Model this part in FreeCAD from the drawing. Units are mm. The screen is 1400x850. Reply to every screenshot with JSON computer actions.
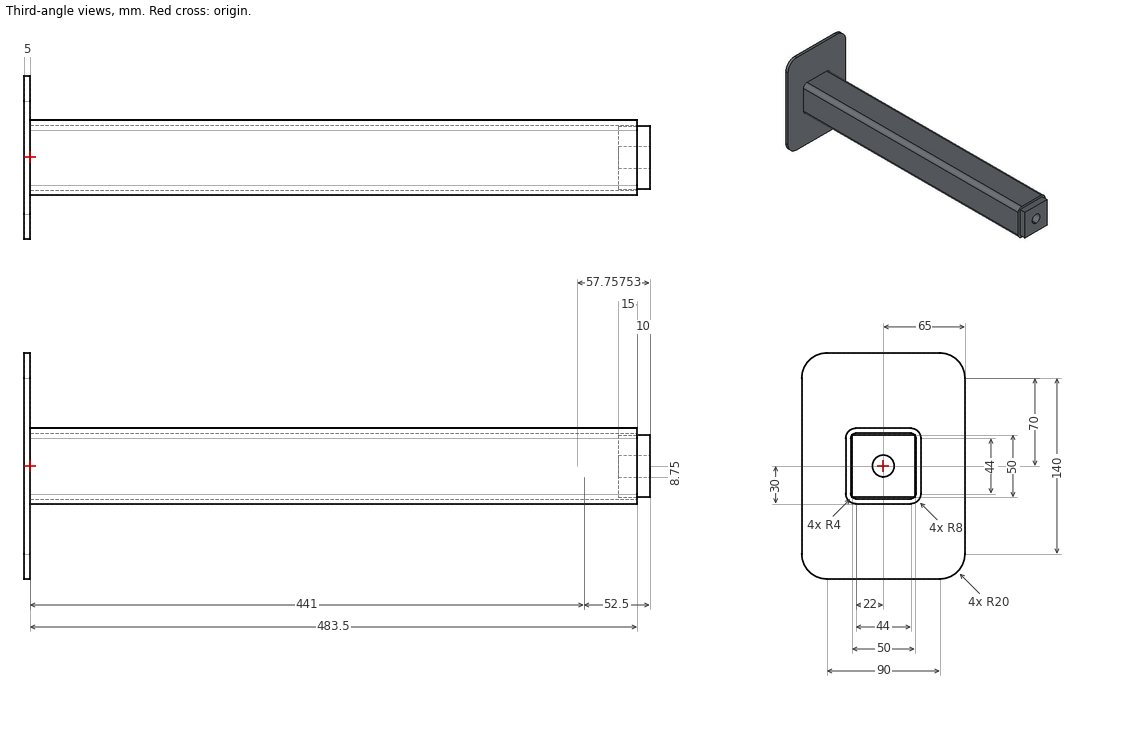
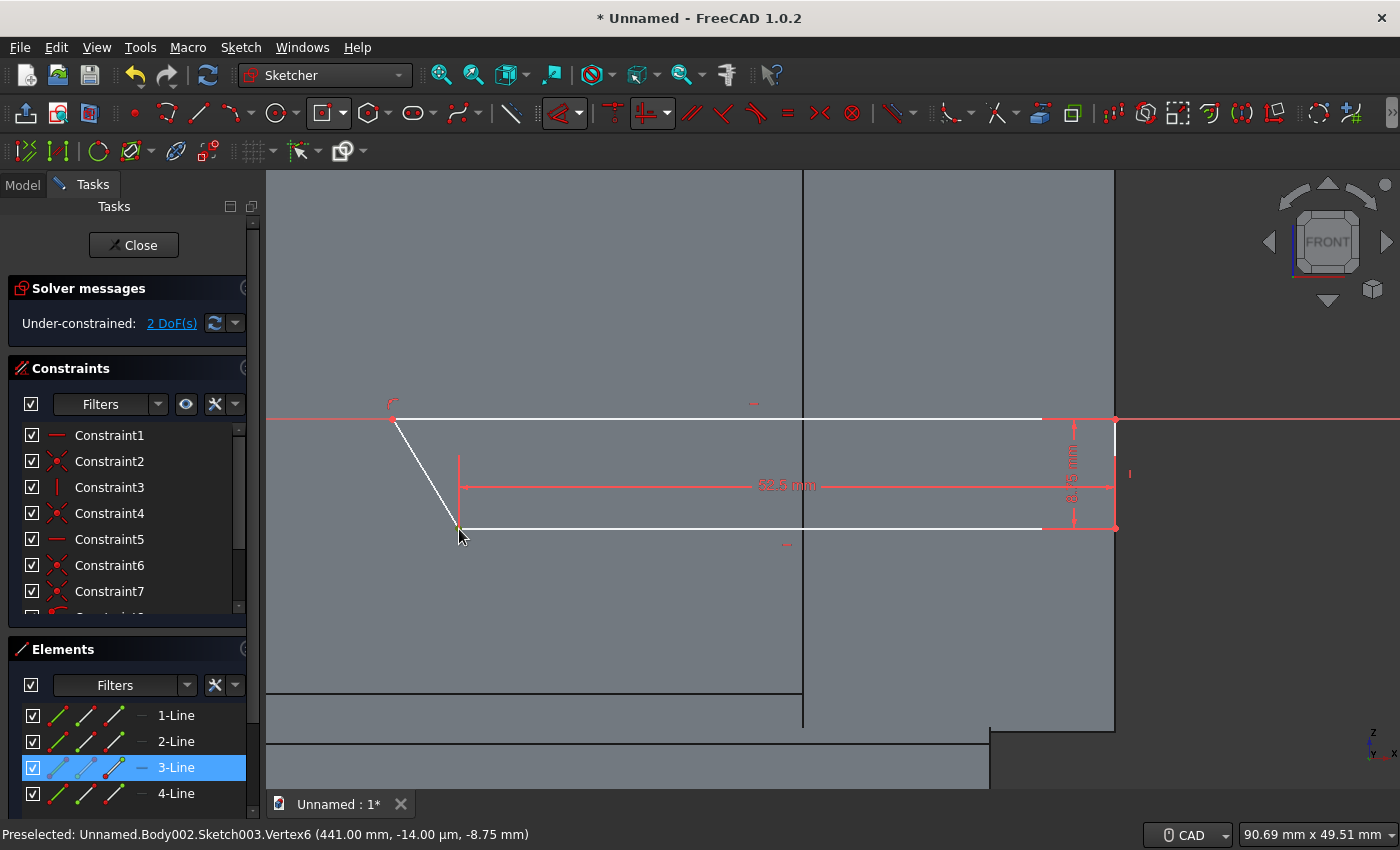
{"action": "left_click", "coordinate": [582, 114]}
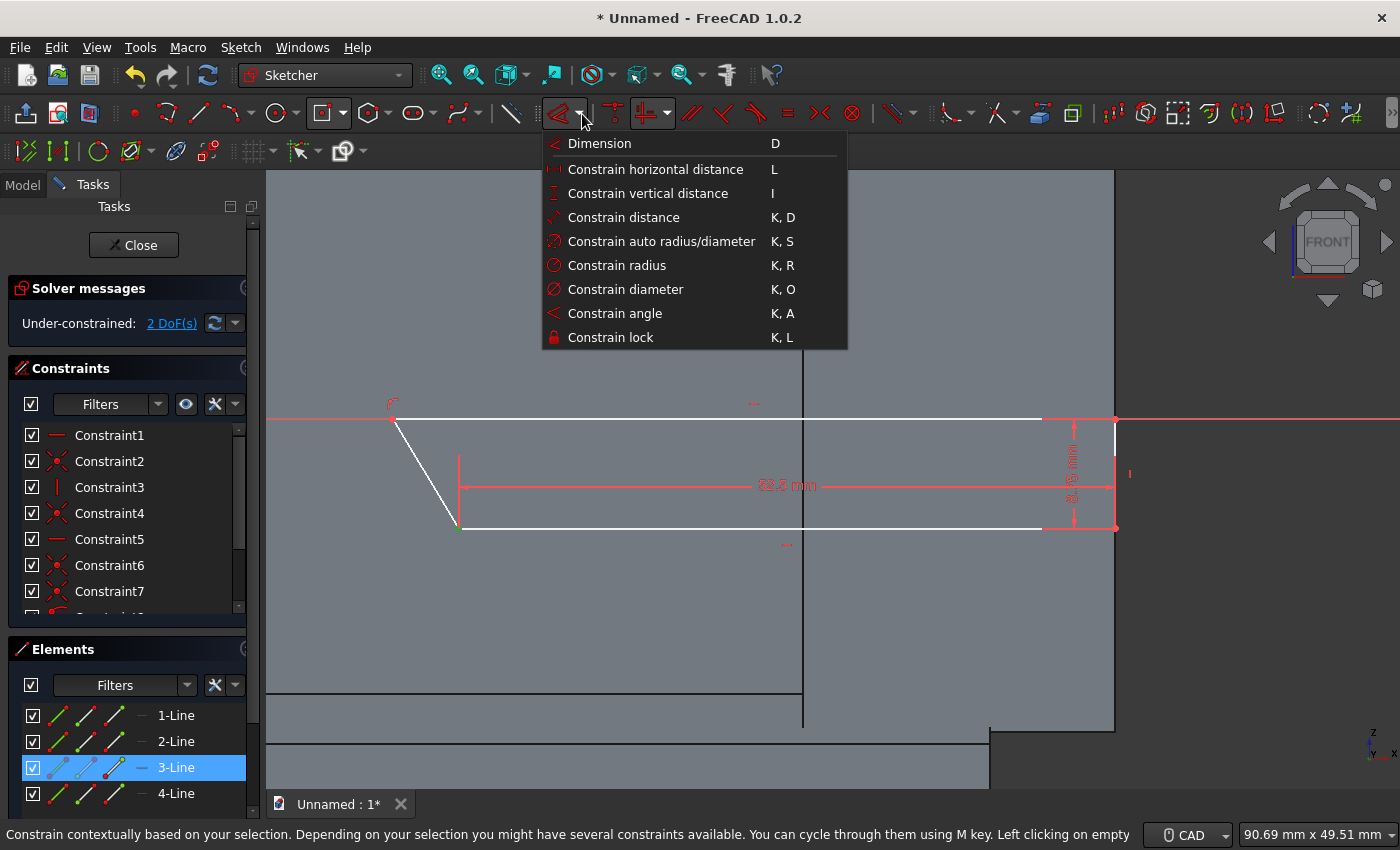
{"action": "left_click", "coordinate": [695, 169]}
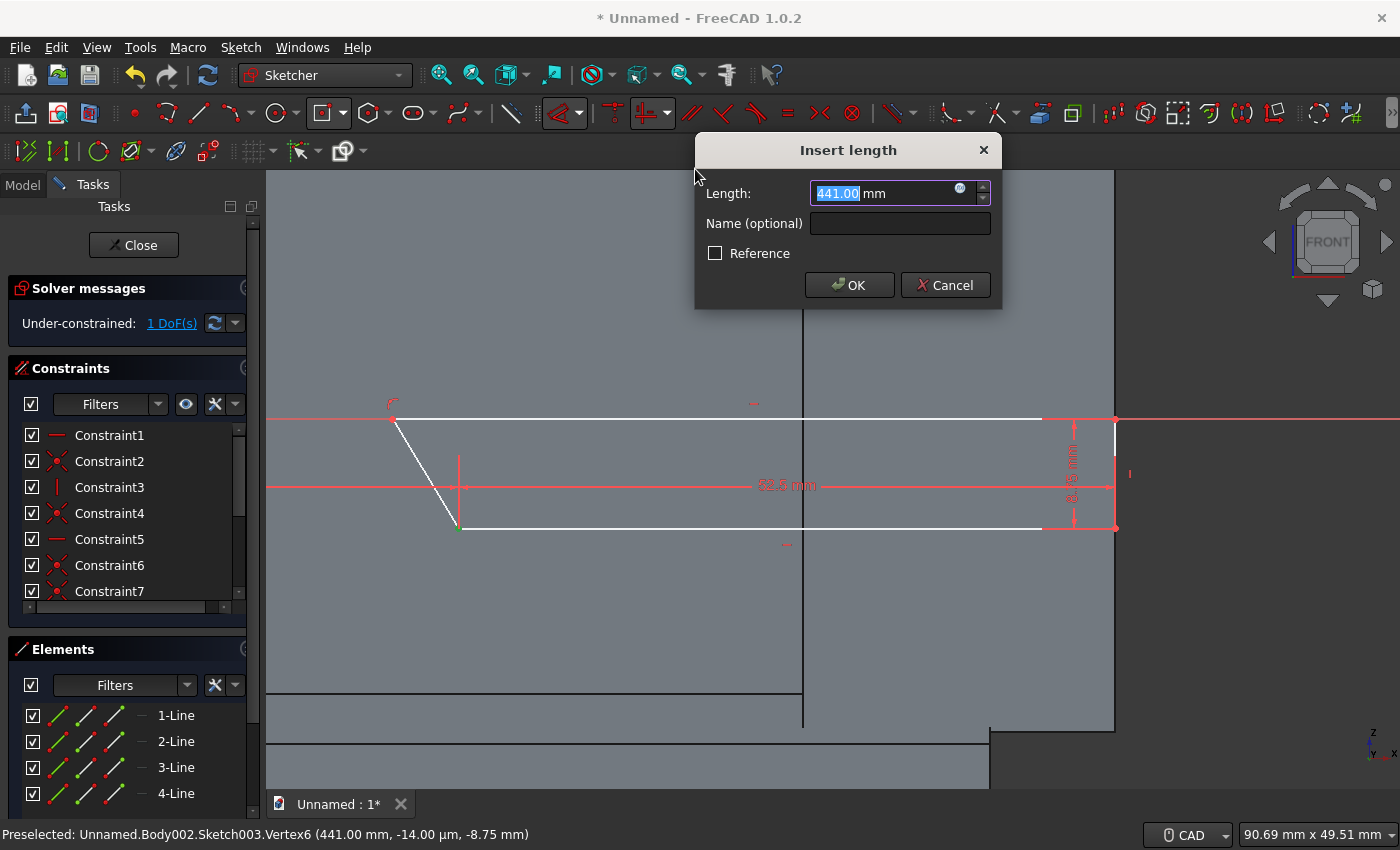
{"action": "type", "text": "441"}
{"action": "key", "text": "Return"}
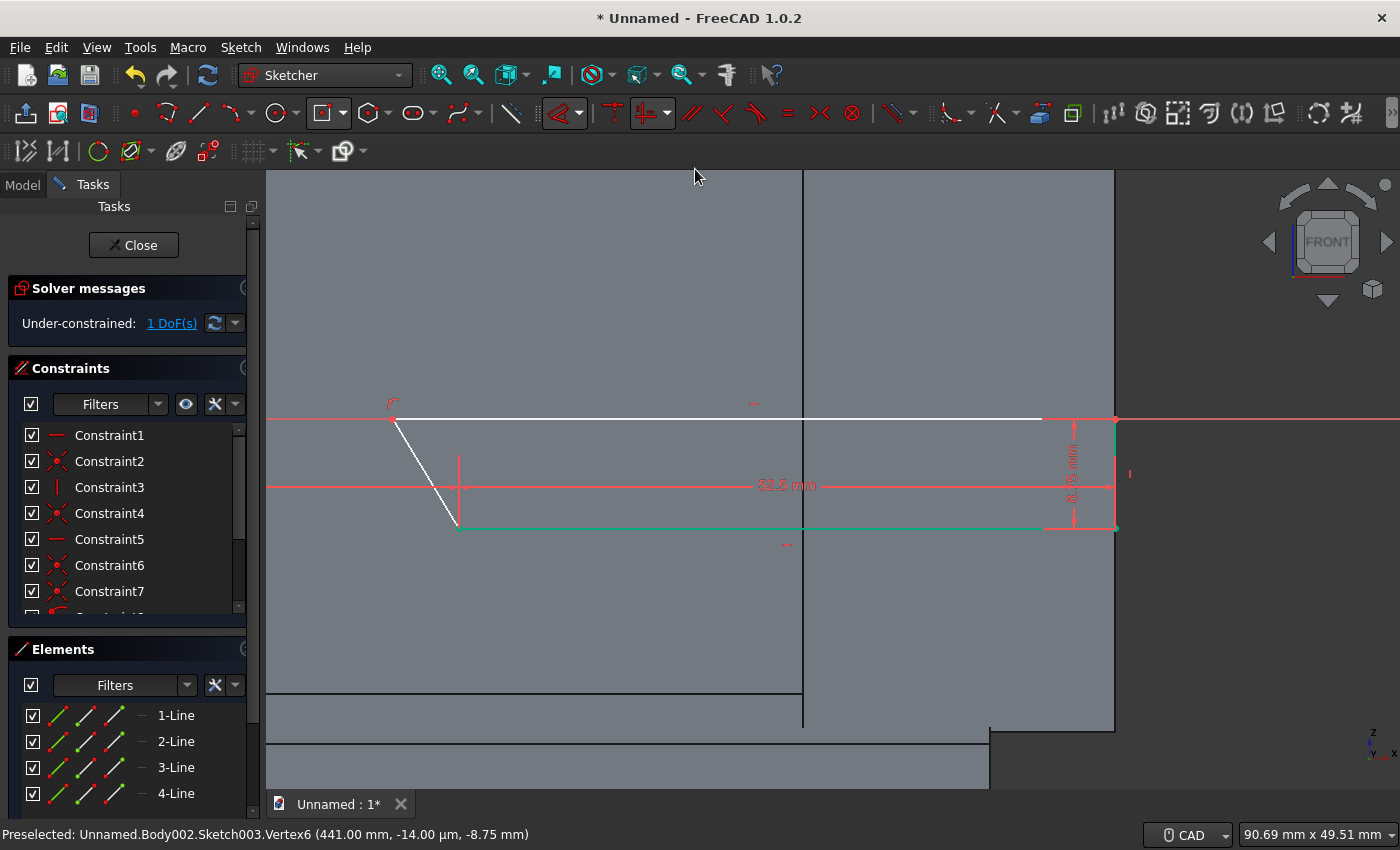
{"action": "left_click", "coordinate": [610, 419]}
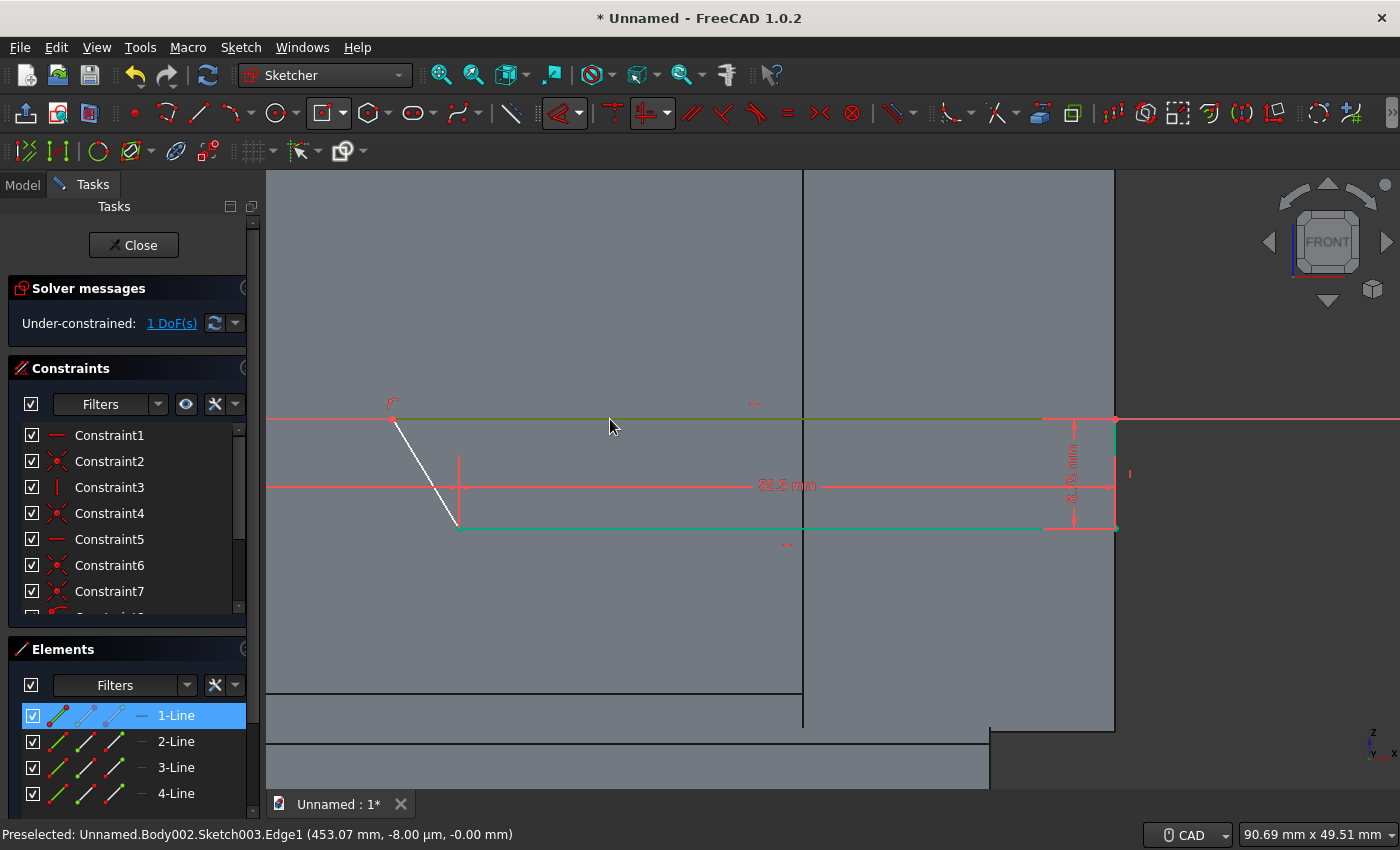
{"action": "left_click", "coordinate": [582, 114]}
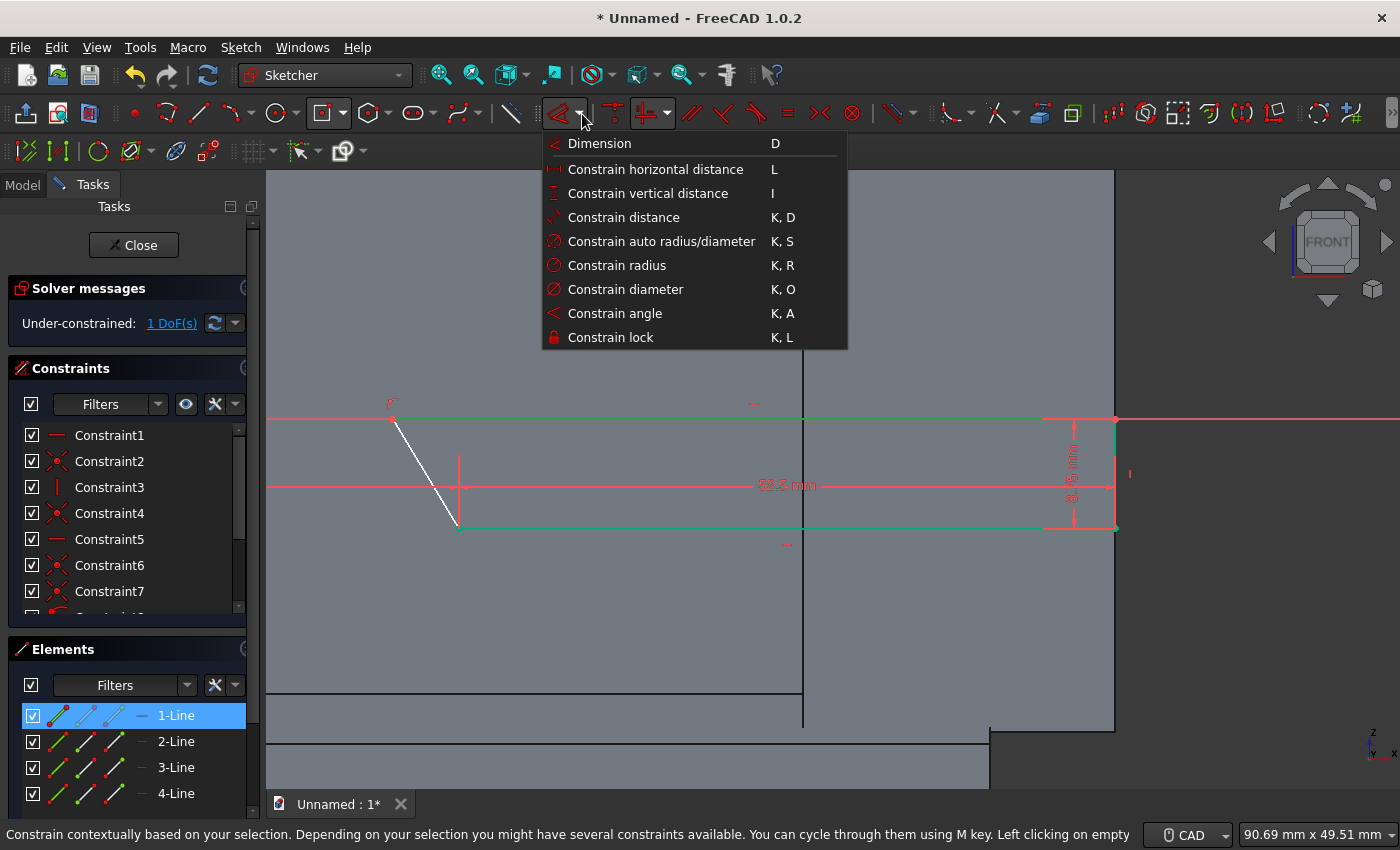
{"action": "left_click", "coordinate": [695, 169]}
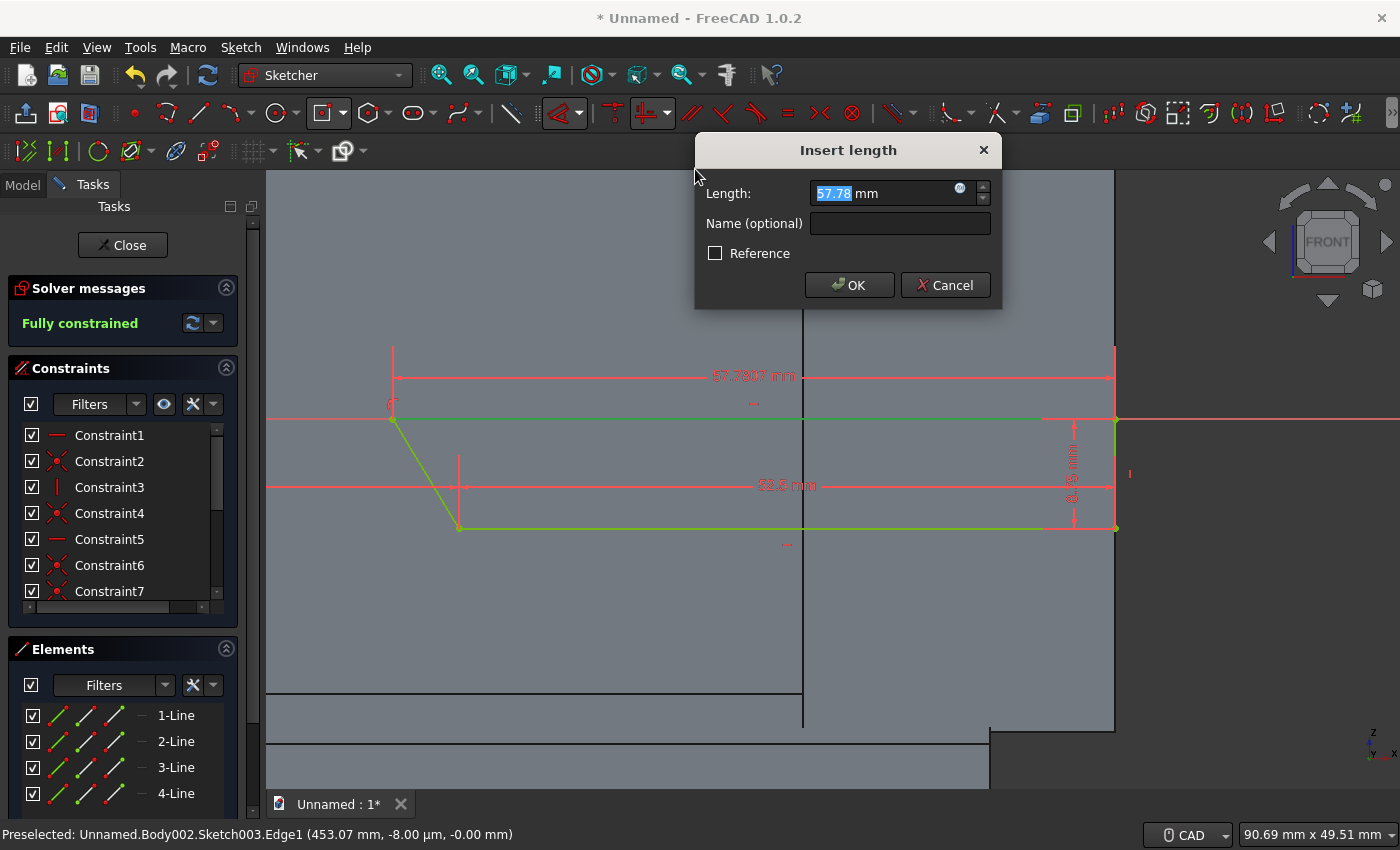
{"action": "type", "text": "57.75753"}
{"action": "key", "text": "Return"}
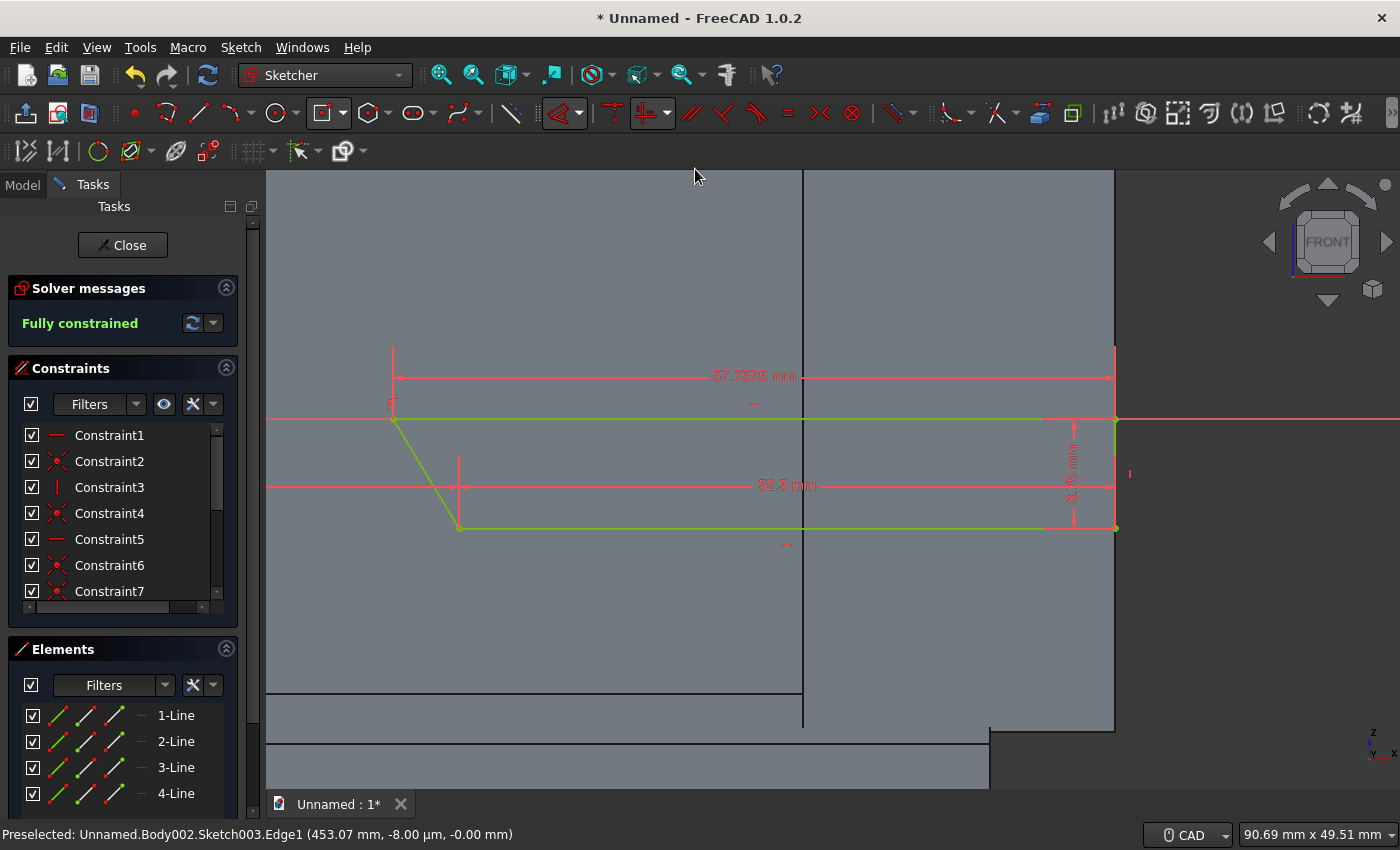
{"action": "left_click", "coordinate": [123, 245]}